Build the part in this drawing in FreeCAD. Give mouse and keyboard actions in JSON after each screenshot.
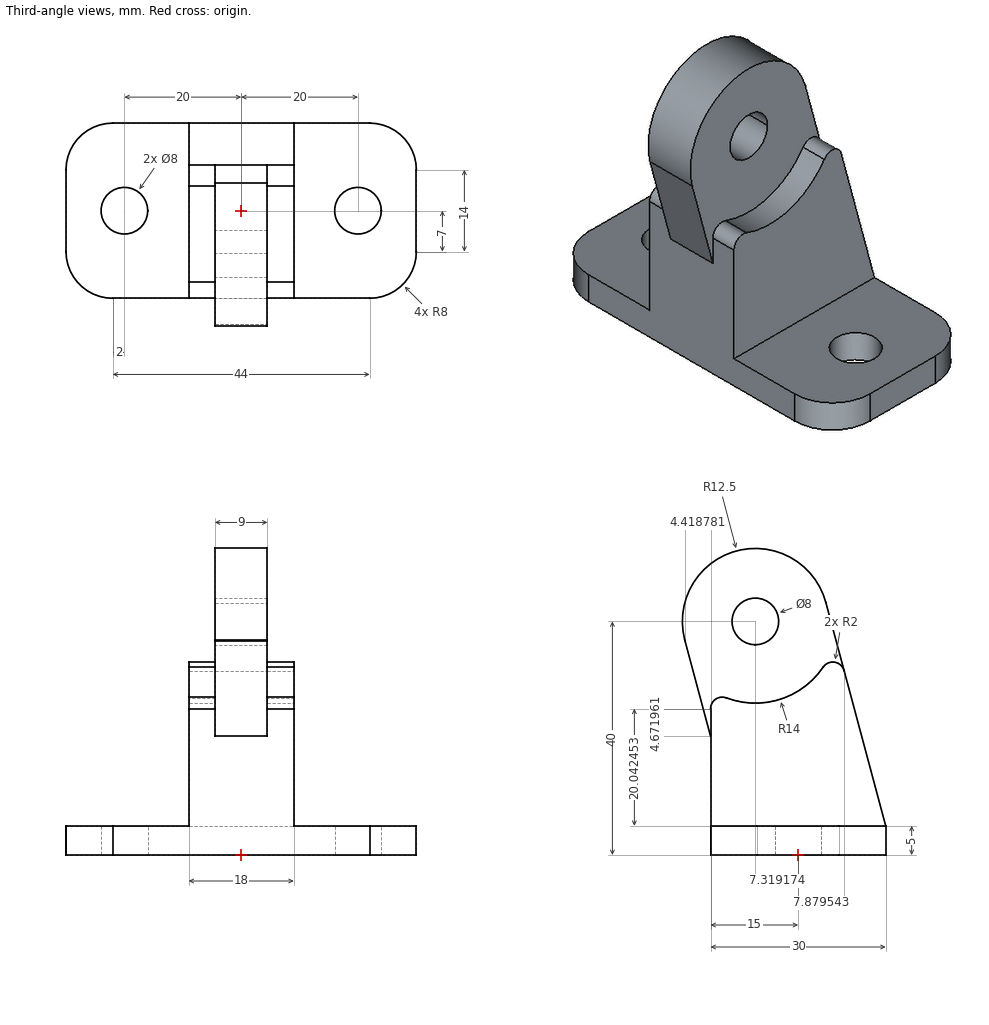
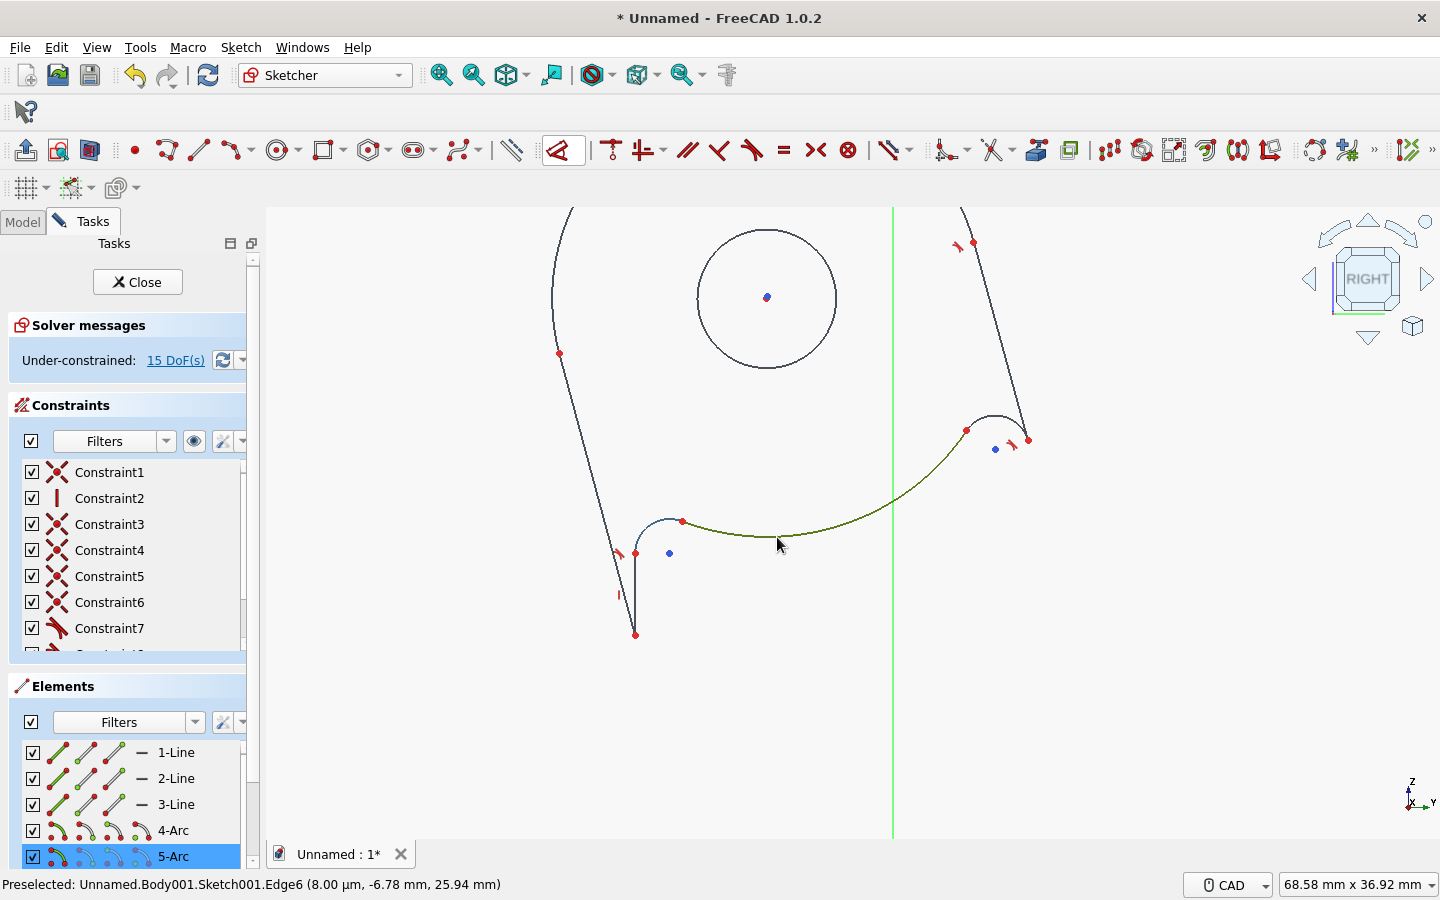
{"action": "key", "text": "t"}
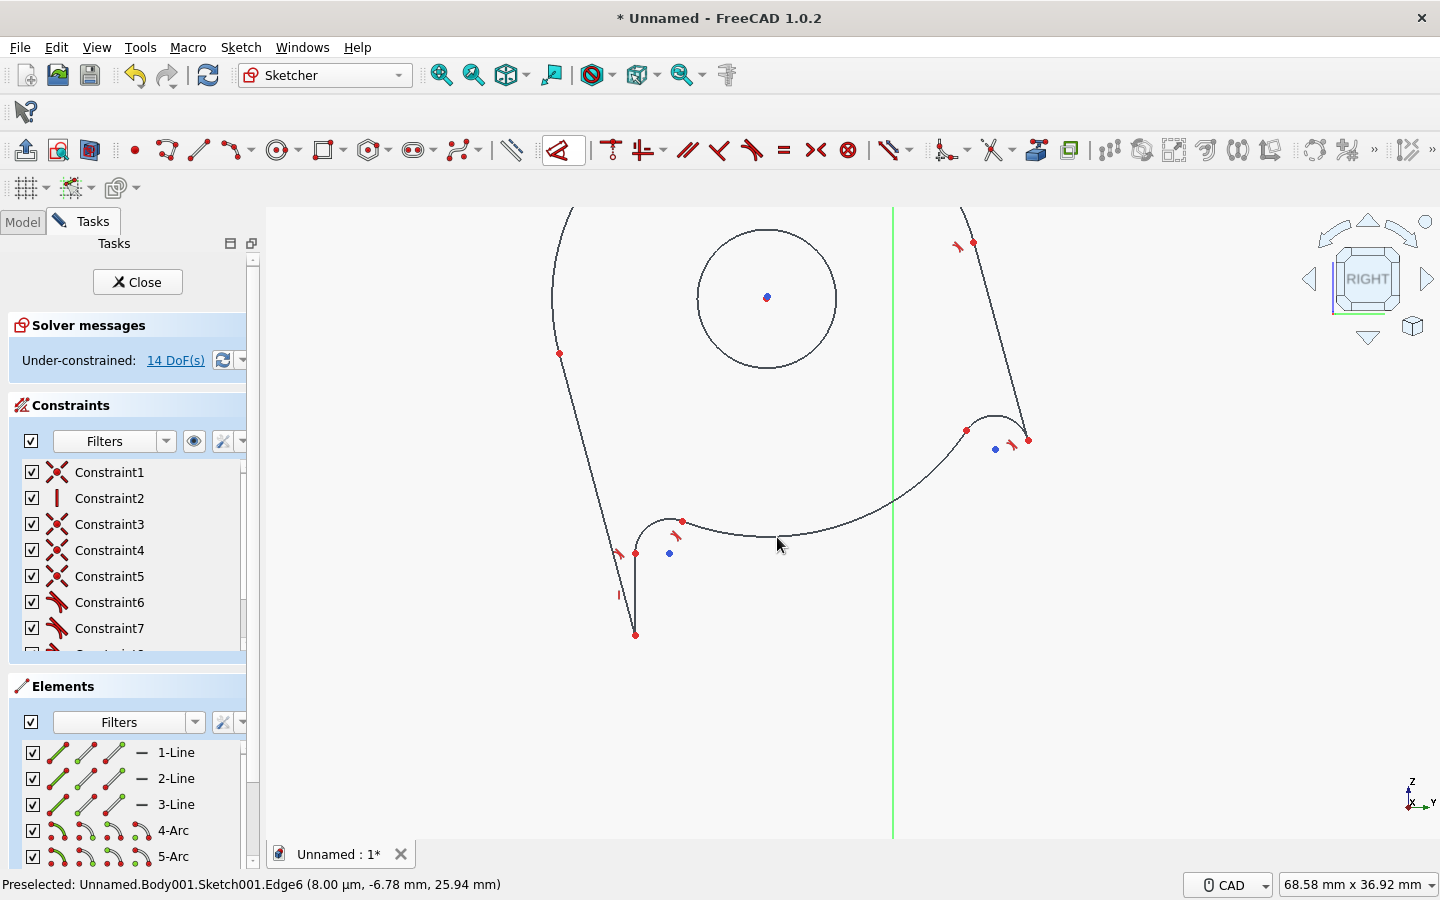
{"action": "left_click", "coordinate": [777, 537]}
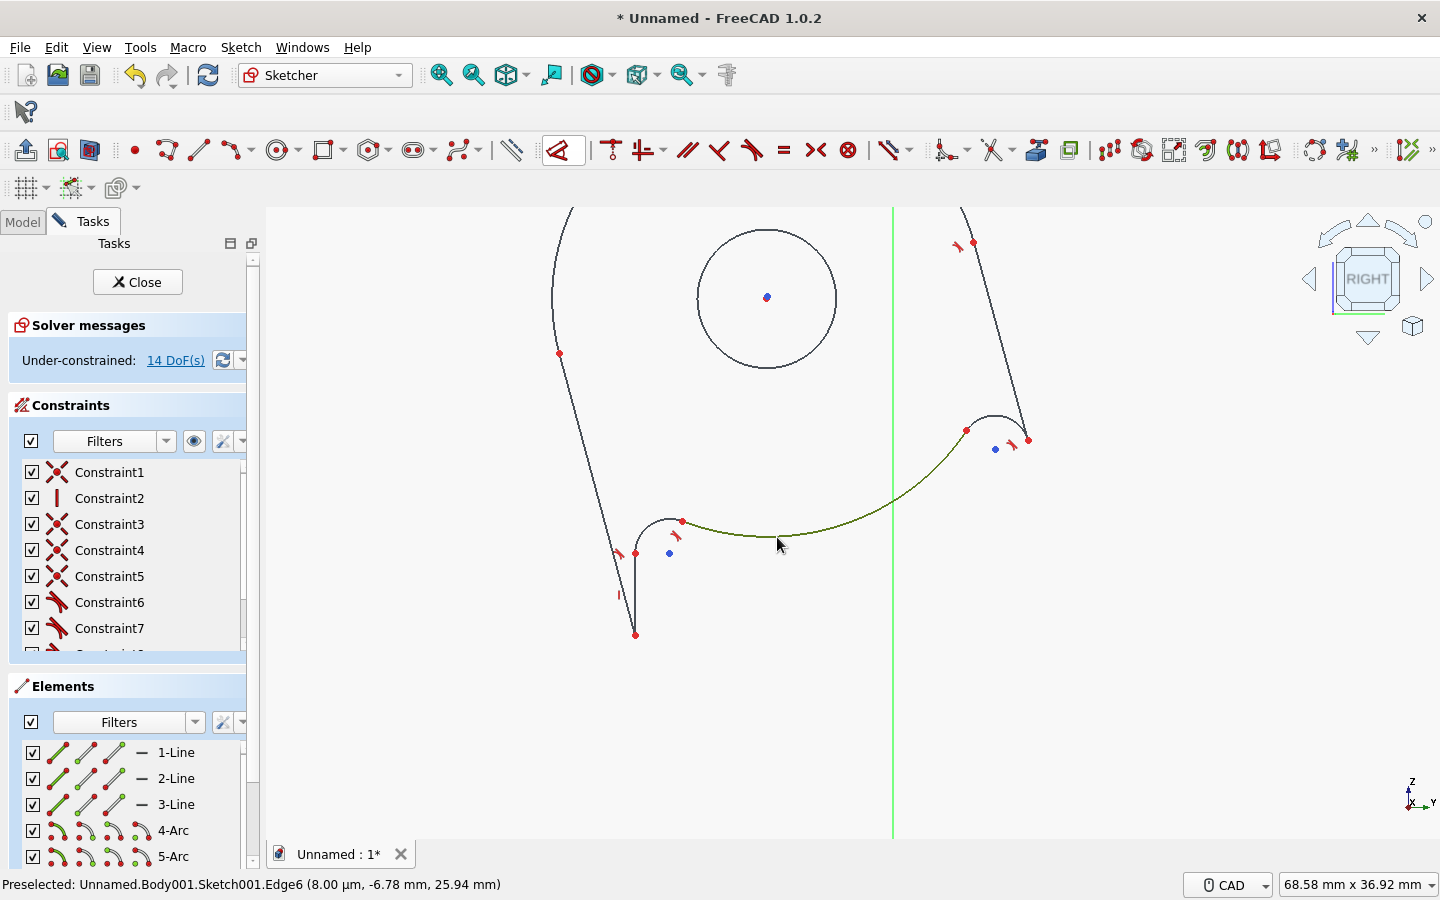
{"action": "left_click", "coordinate": [985, 417]}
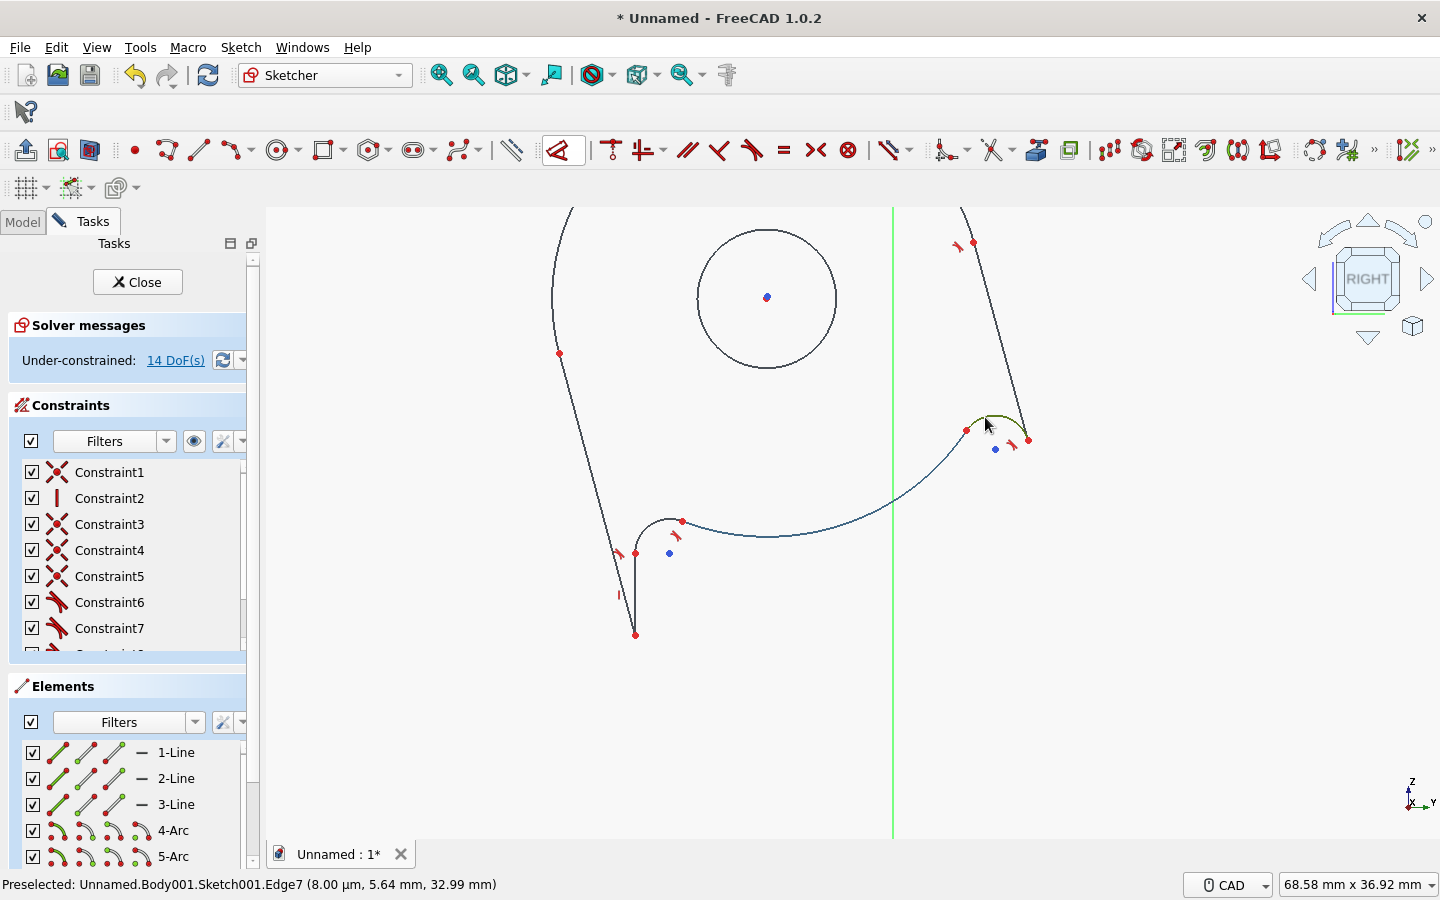
{"action": "key", "text": "t"}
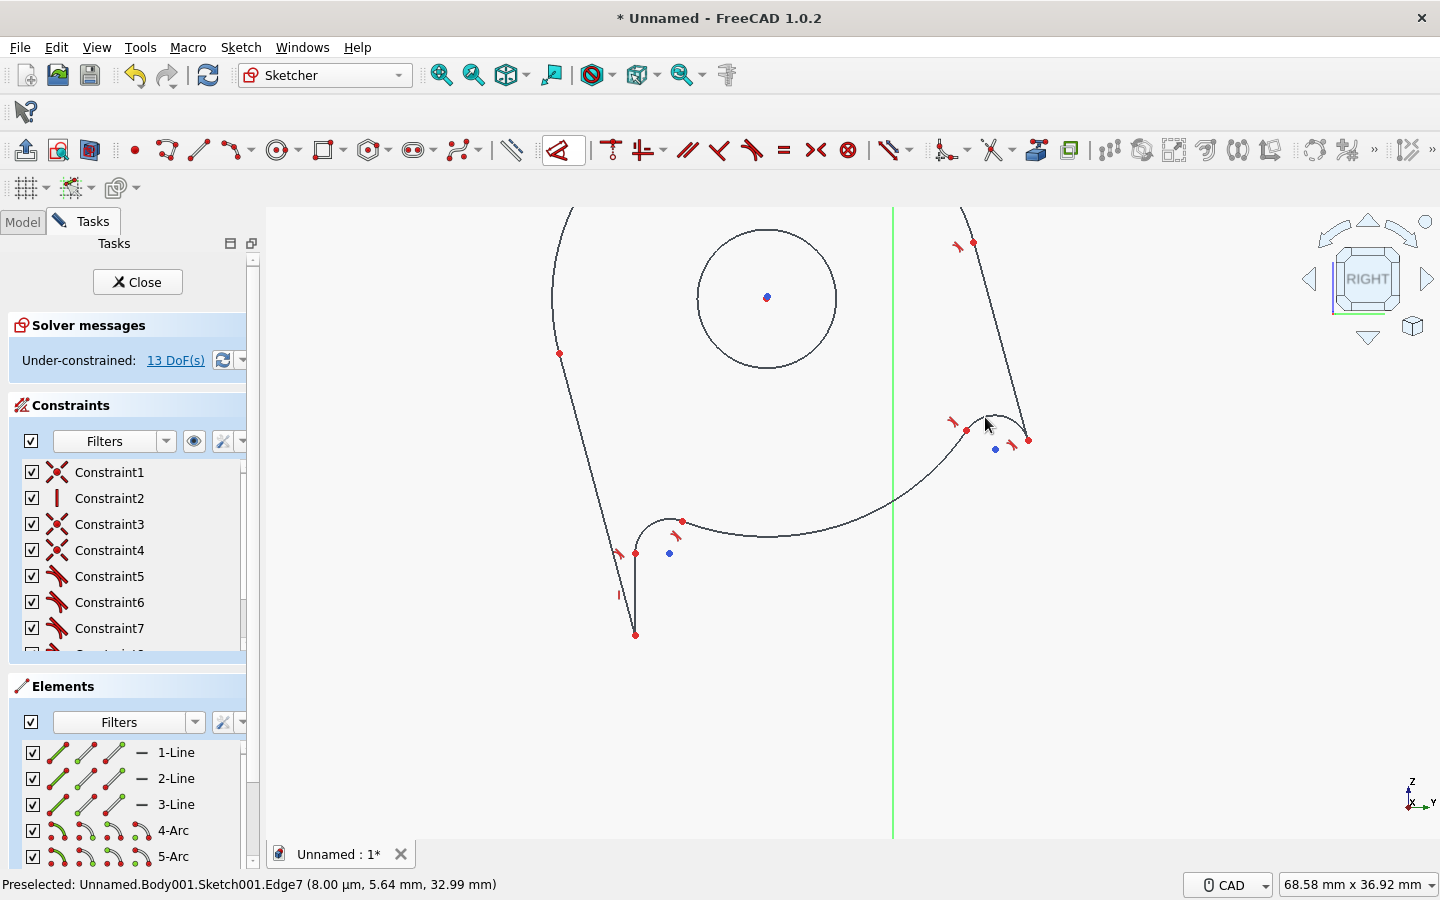
{"action": "left_click", "coordinate": [816, 250]}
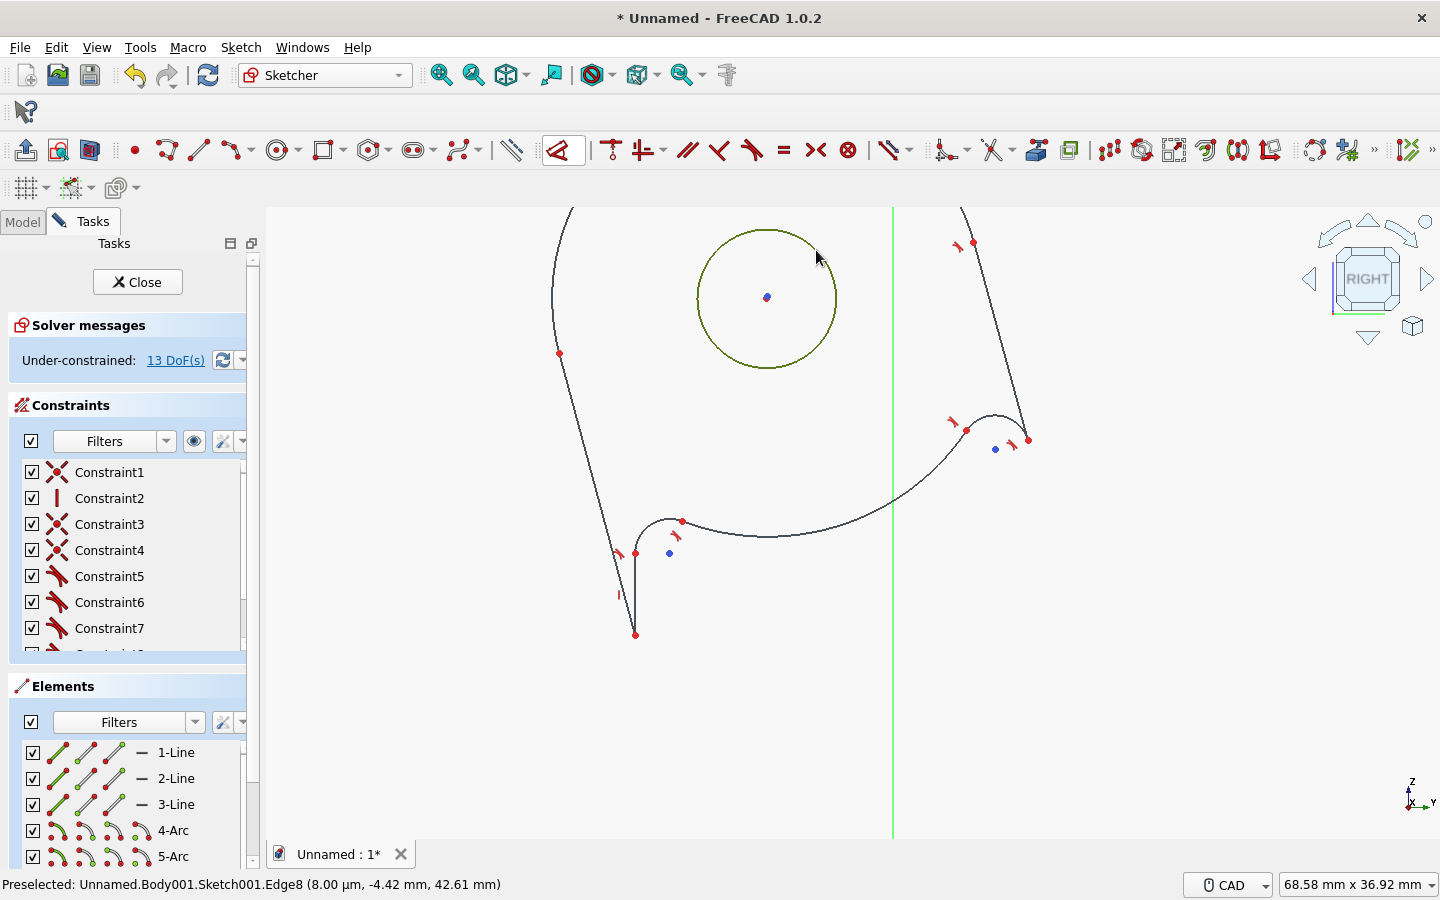
{"action": "left_click", "coordinate": [777, 537]}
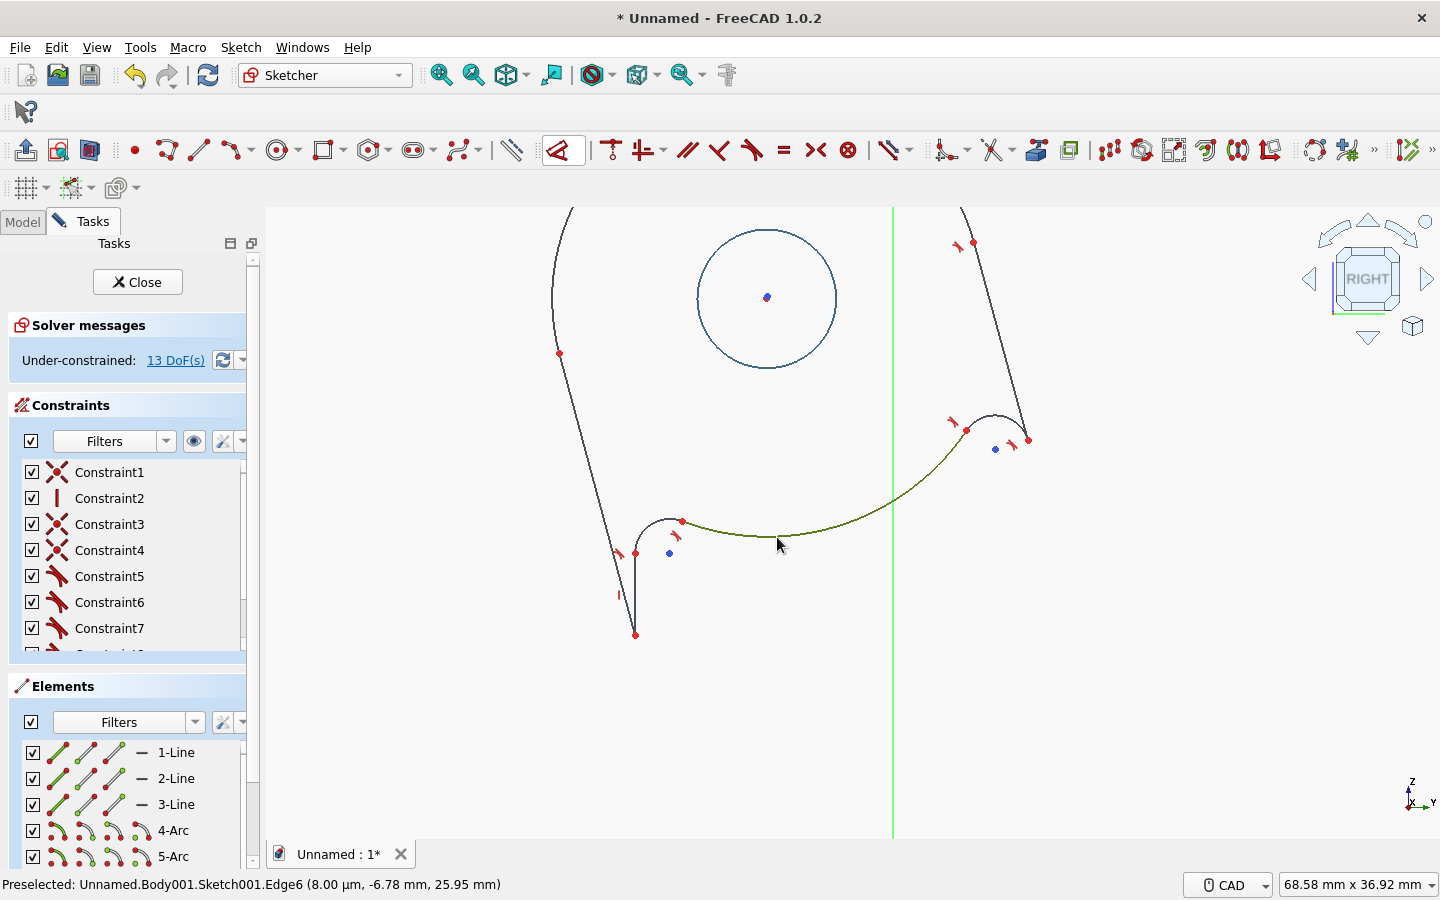
{"action": "left_click", "coordinate": [612, 150]}